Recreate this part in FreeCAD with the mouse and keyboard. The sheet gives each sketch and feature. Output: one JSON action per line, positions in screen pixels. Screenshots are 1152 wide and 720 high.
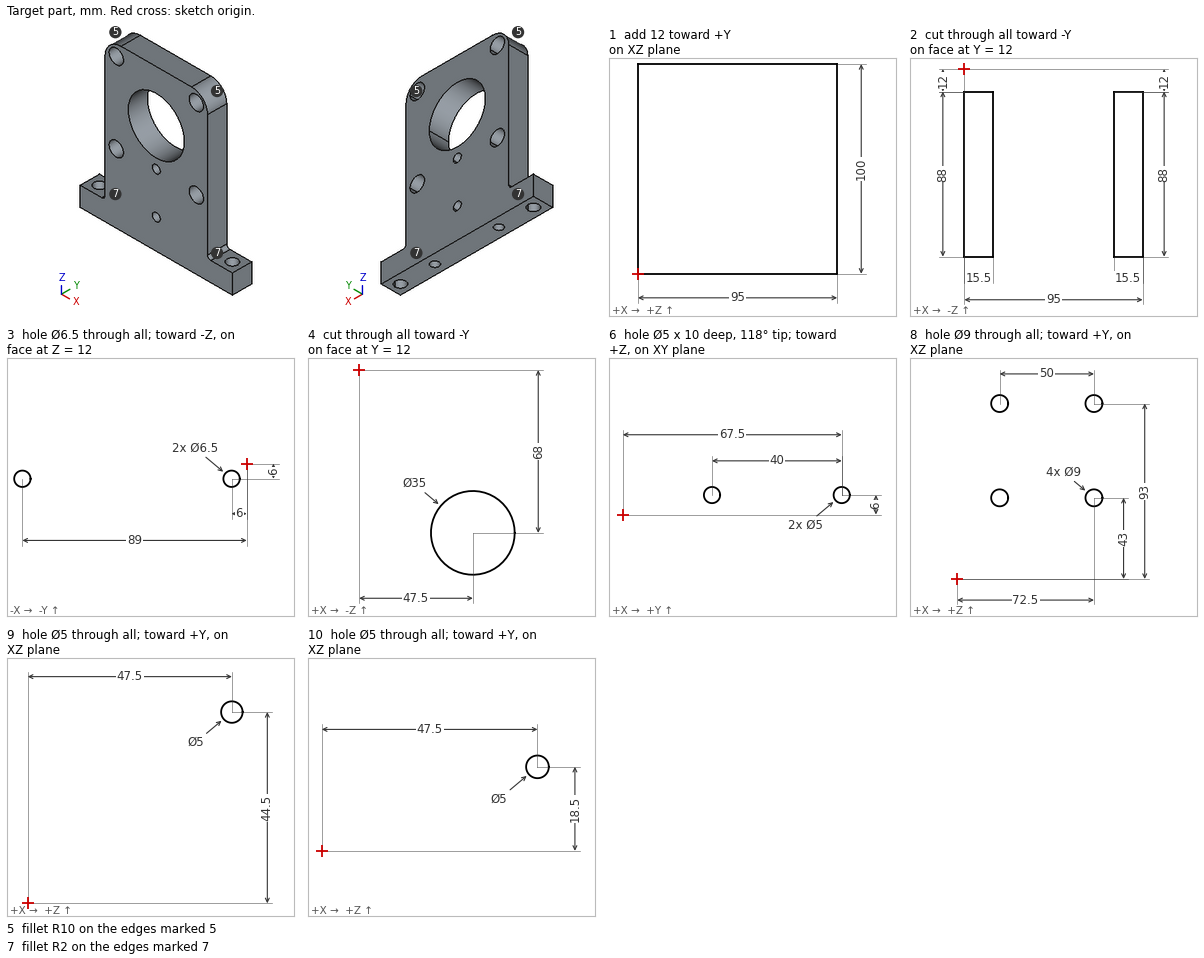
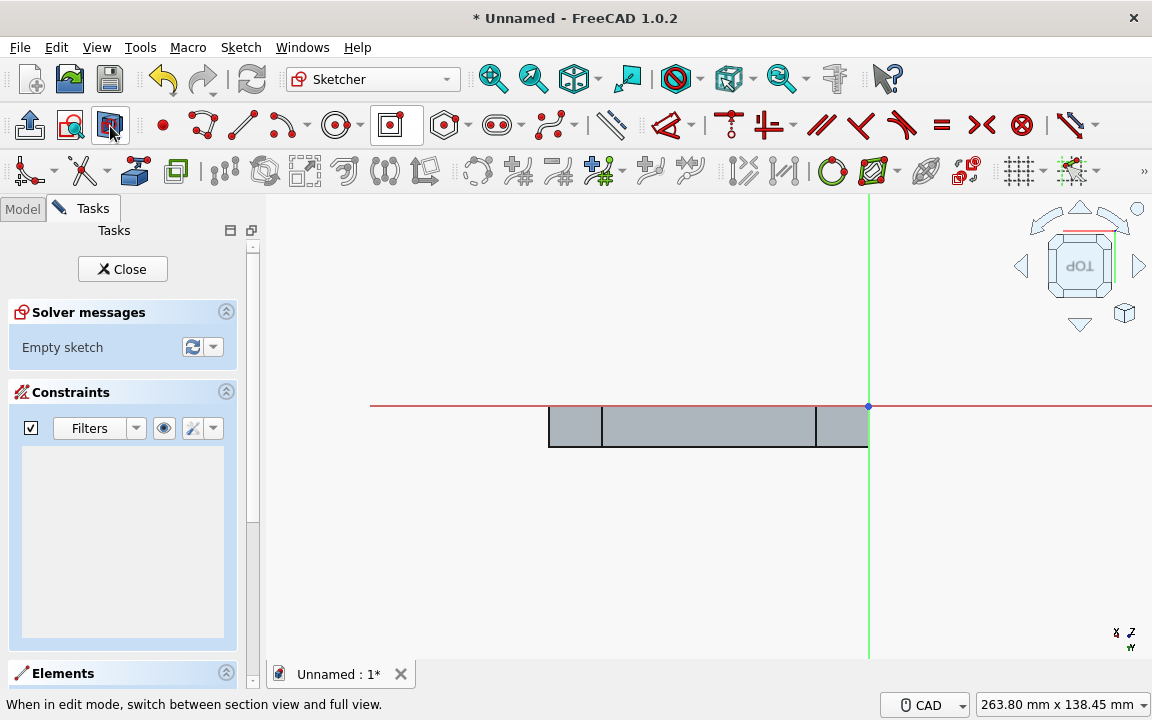
{"action": "scroll", "coordinate": [862, 412], "scroll_direction": "up", "scroll_amount": 2}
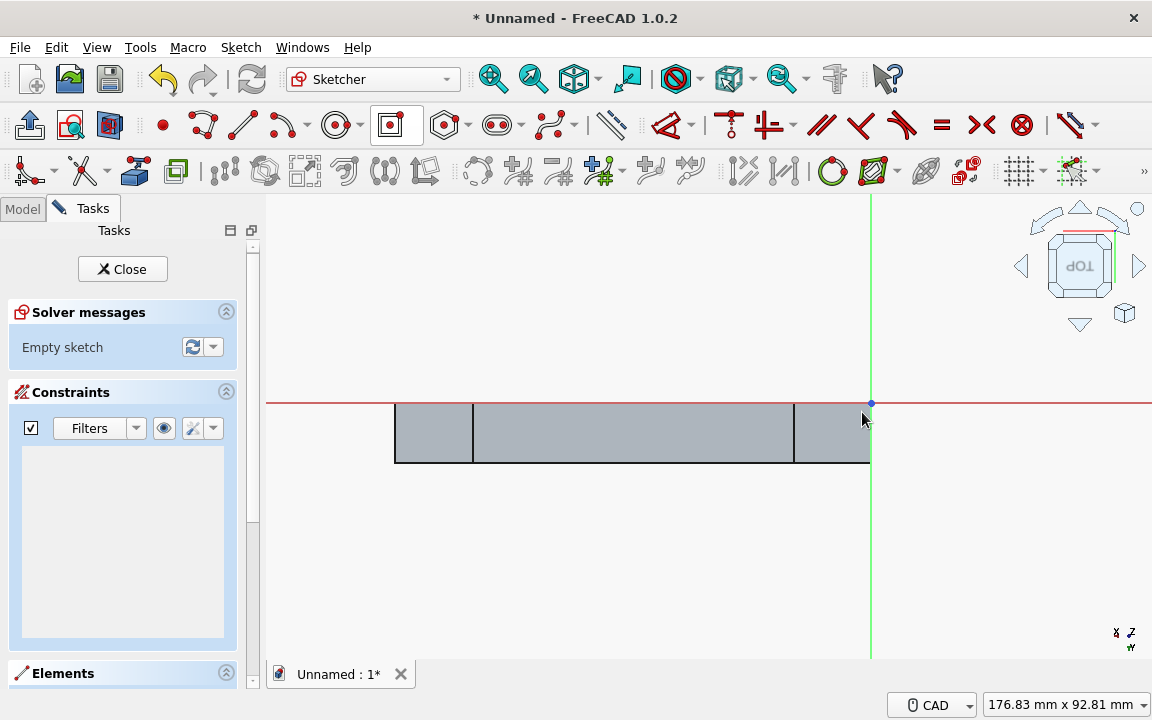
{"action": "left_click", "coordinate": [336, 126]}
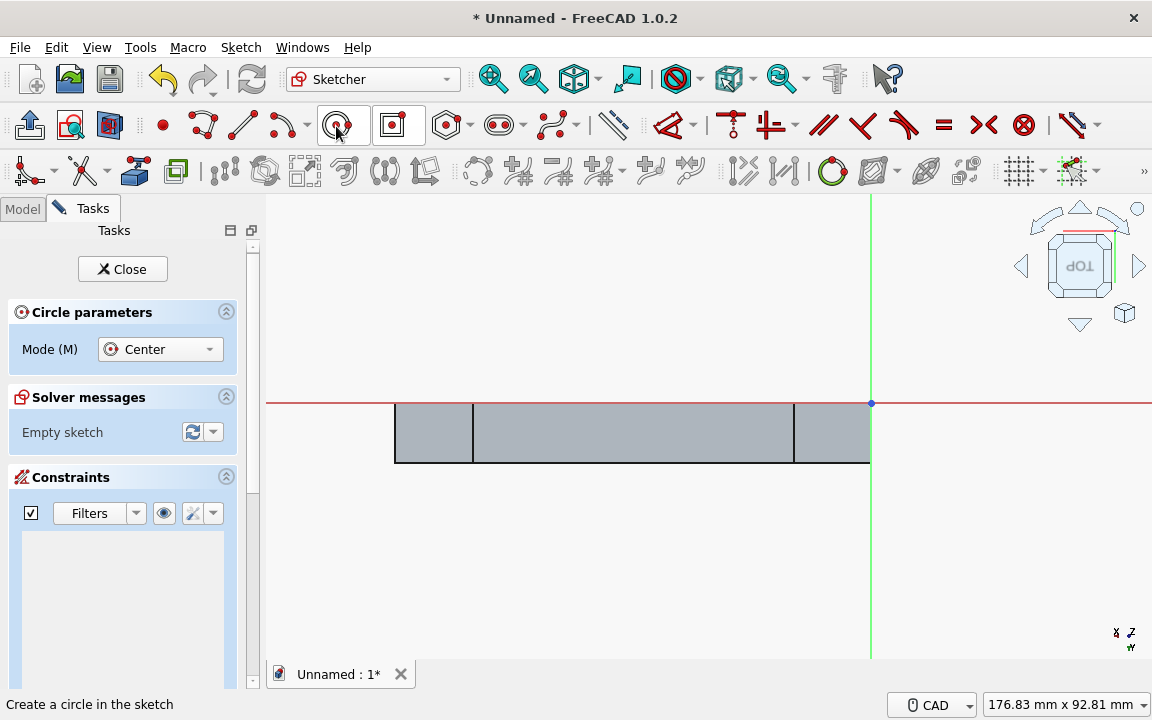
{"action": "scroll", "coordinate": [841, 433], "scroll_direction": "up", "scroll_amount": 2}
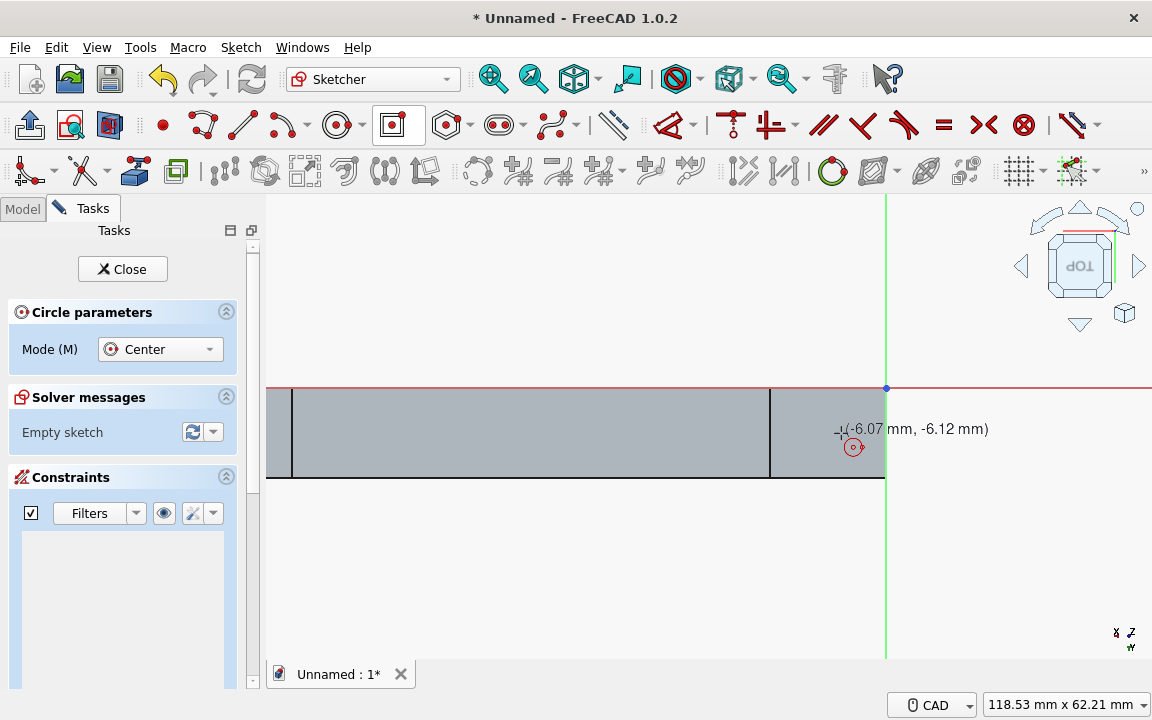
{"action": "left_click", "coordinate": [841, 433]}
{"action": "left_click", "coordinate": [858, 416]}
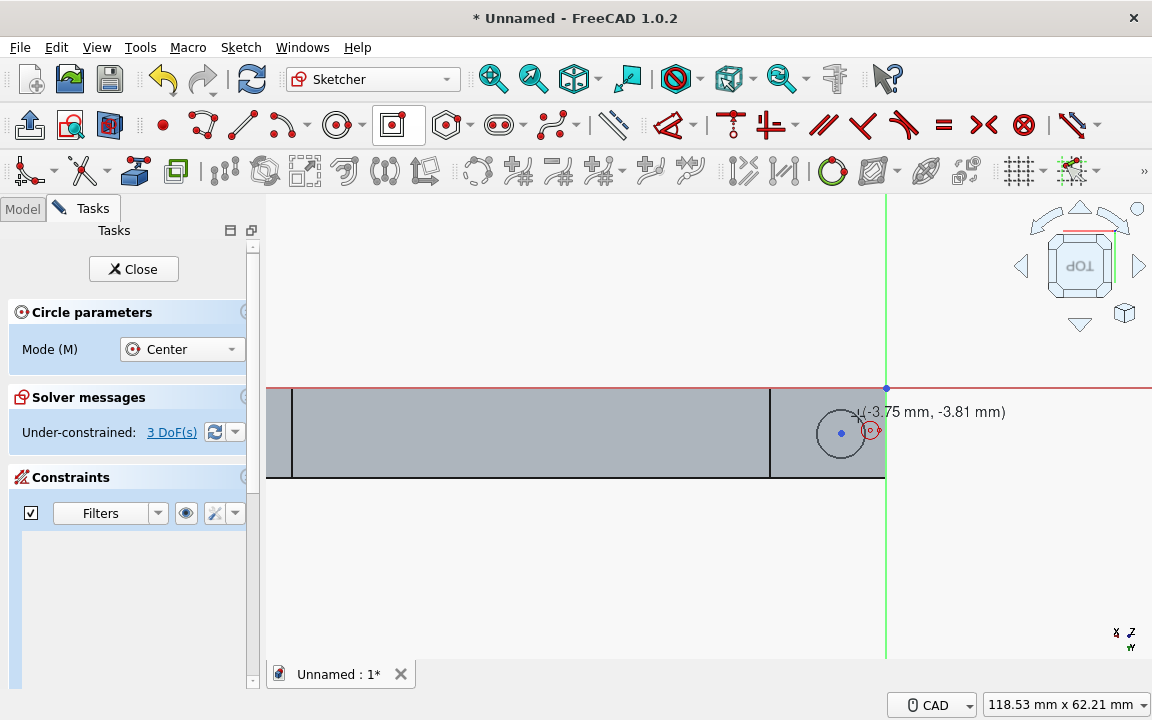
{"action": "scroll", "coordinate": [842, 433], "scroll_direction": "down", "scroll_amount": 2}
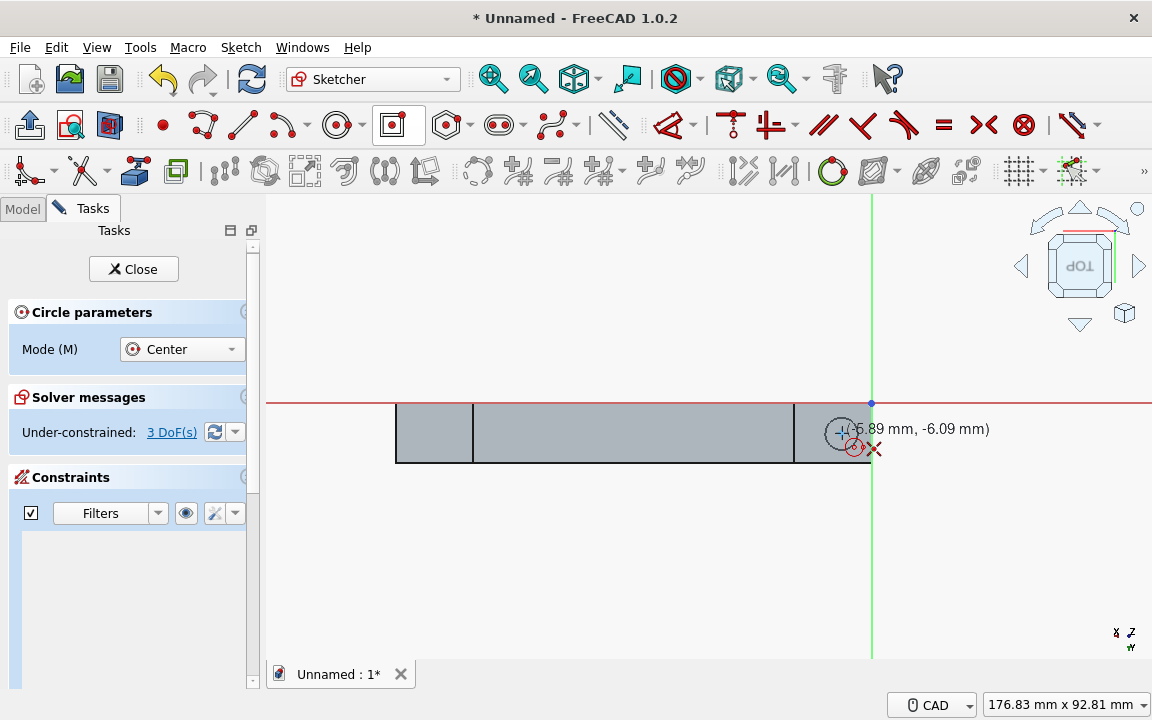
{"action": "scroll", "coordinate": [426, 433], "scroll_direction": "up", "scroll_amount": 2}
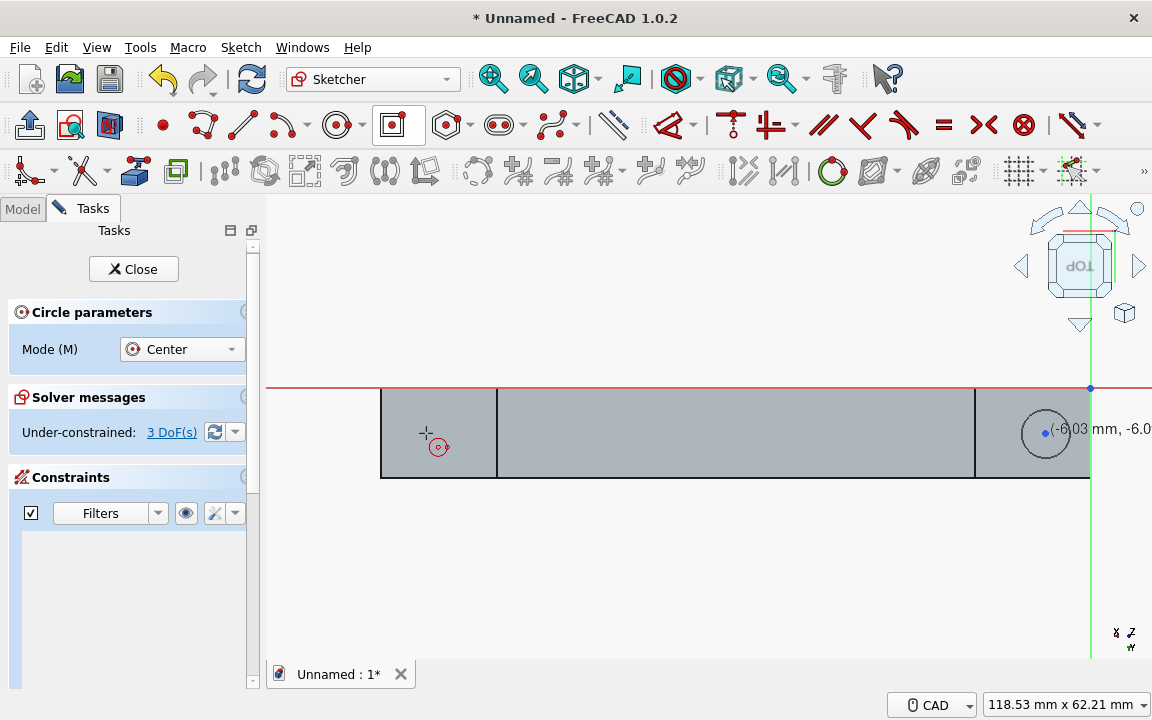
{"action": "left_click", "coordinate": [426, 433]}
{"action": "left_click", "coordinate": [443, 416]}
{"action": "key", "text": "Escape"}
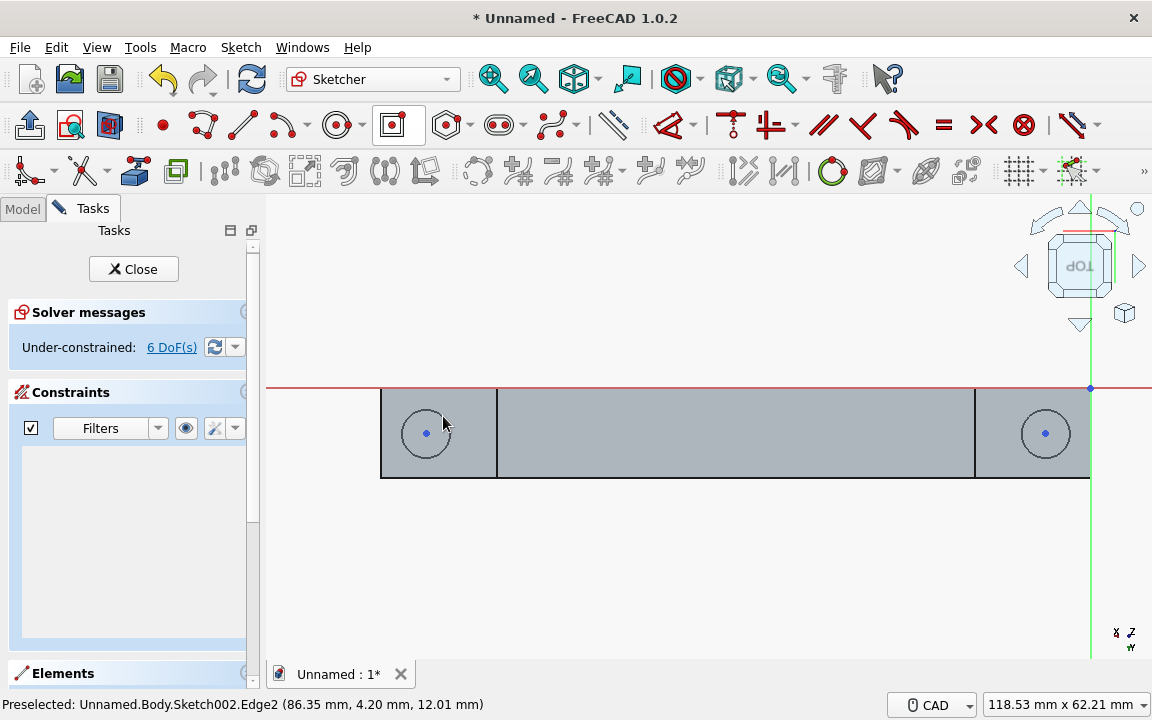
{"action": "scroll", "coordinate": [426, 433], "scroll_direction": "down", "scroll_amount": 2}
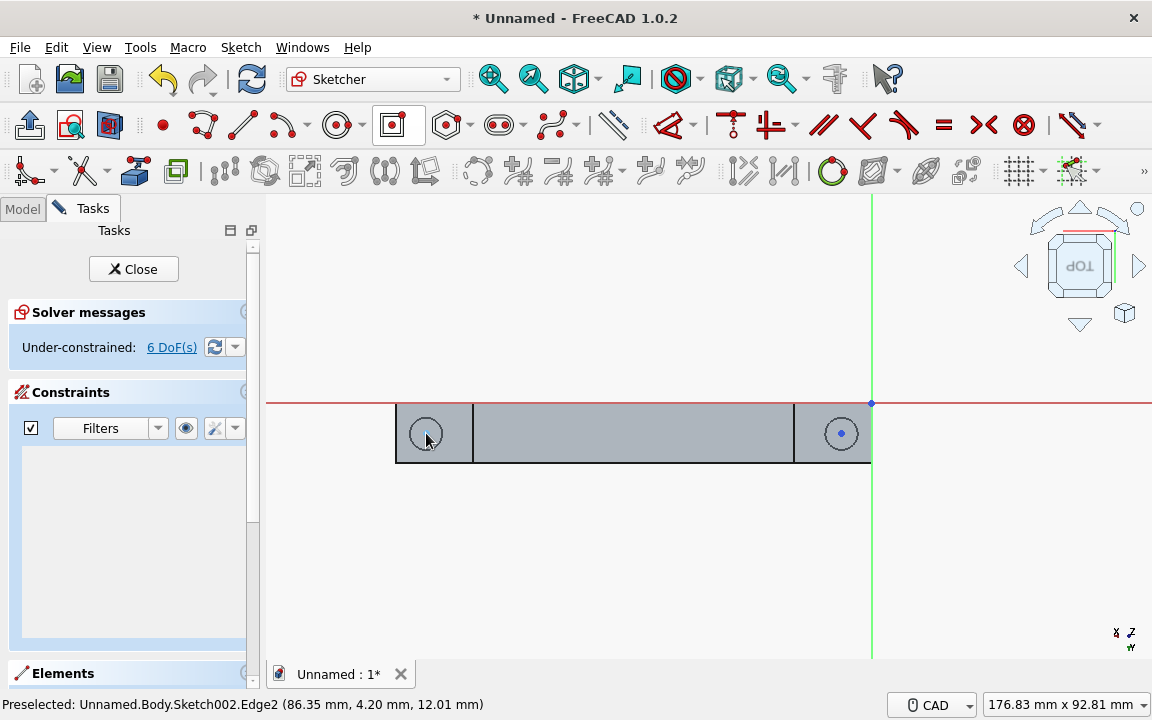
{"action": "left_click", "coordinate": [853, 422]}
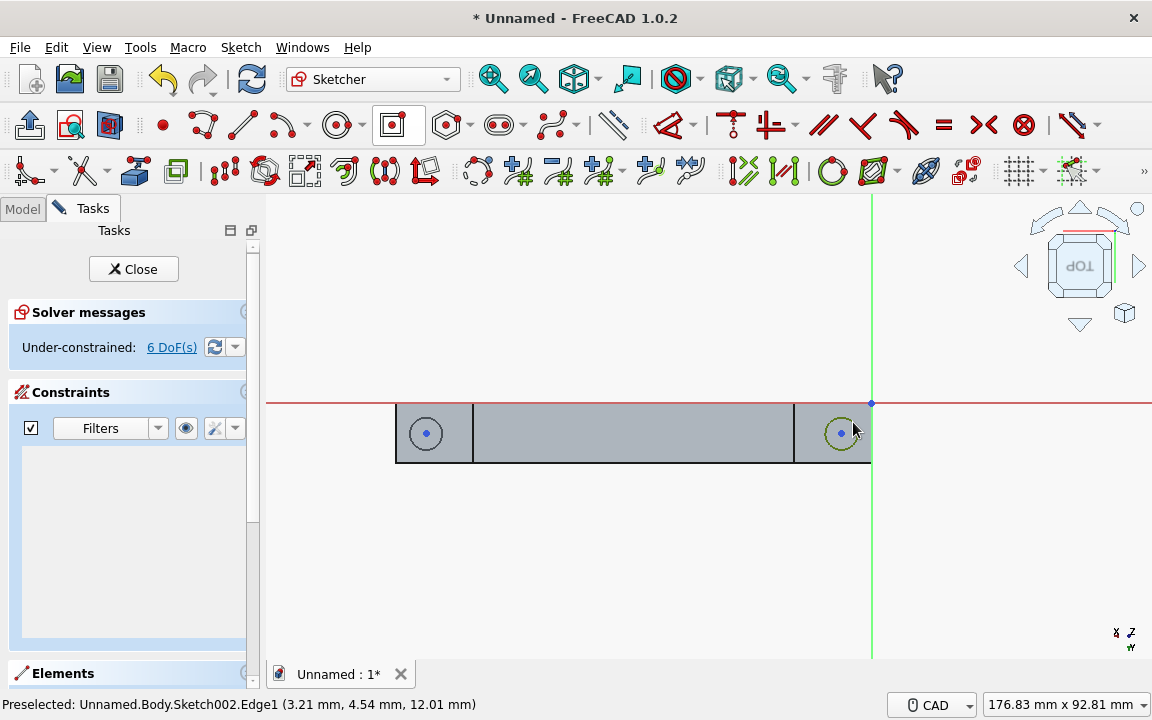
{"action": "left_click", "coordinate": [437, 422]}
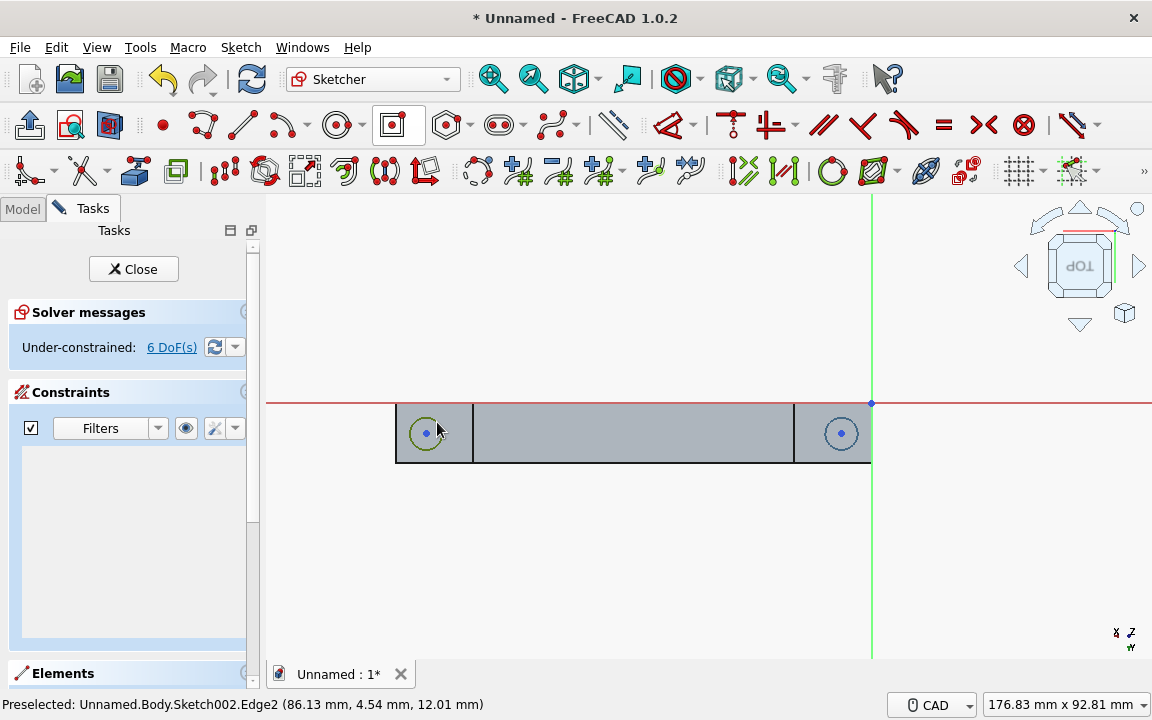
{"action": "left_click", "coordinate": [944, 126]}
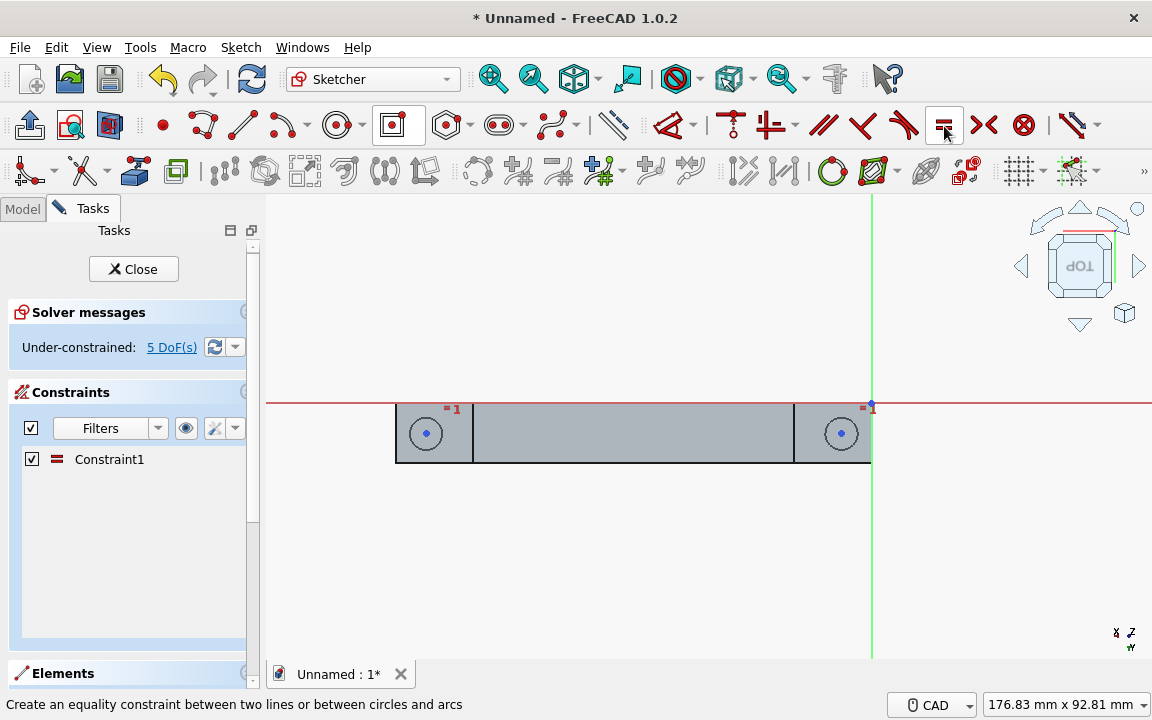
{"action": "left_click", "coordinate": [842, 434]}